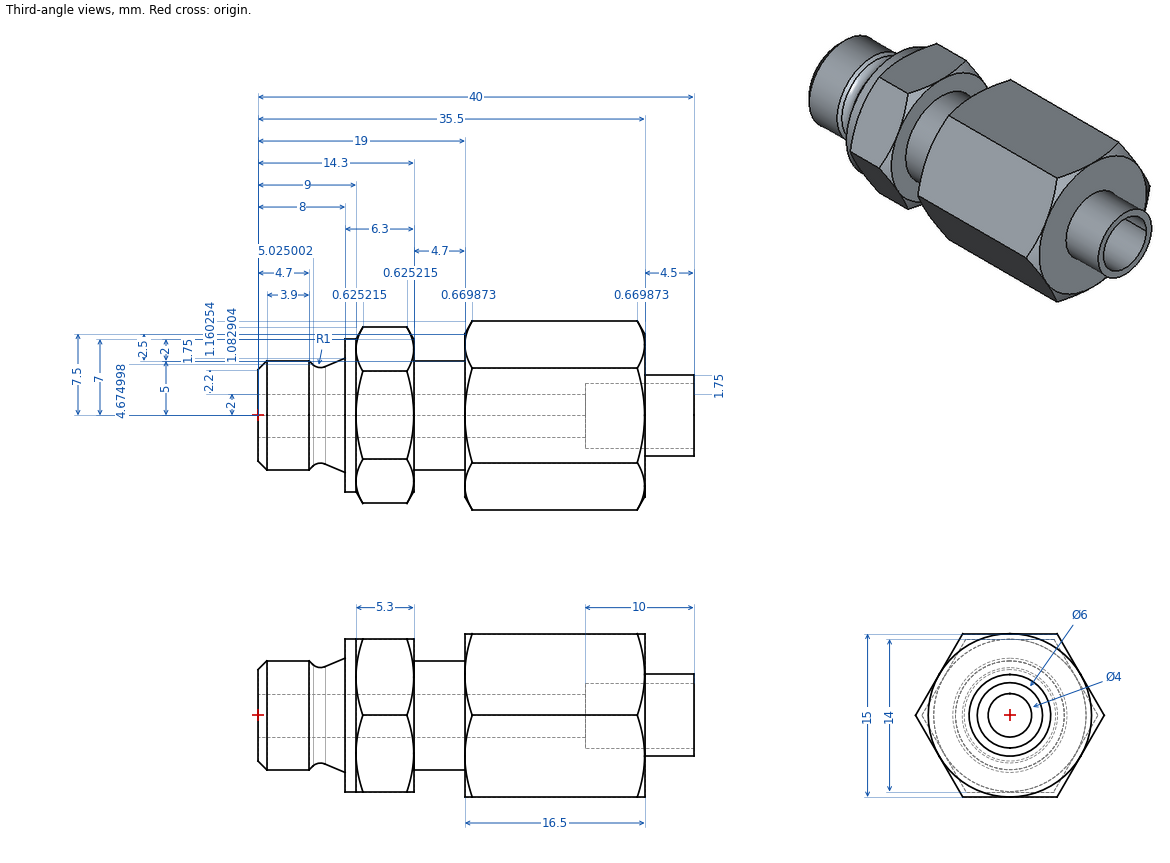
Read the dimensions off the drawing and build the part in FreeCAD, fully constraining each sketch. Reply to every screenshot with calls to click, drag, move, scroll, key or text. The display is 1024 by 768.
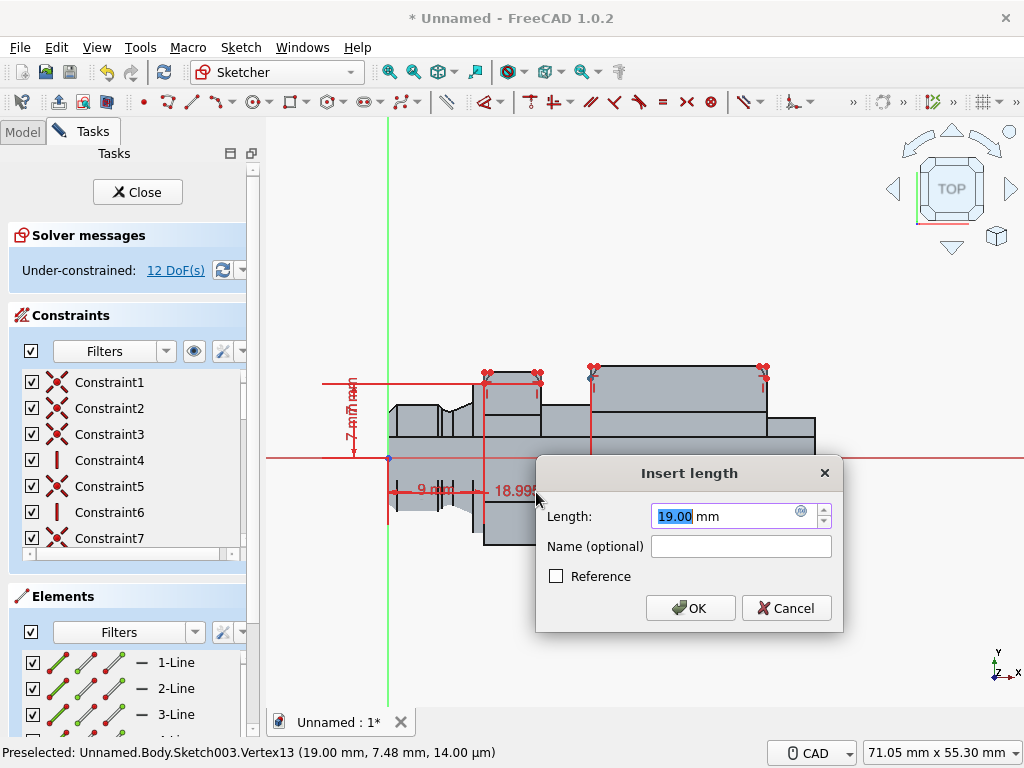
text(19)
key(Return)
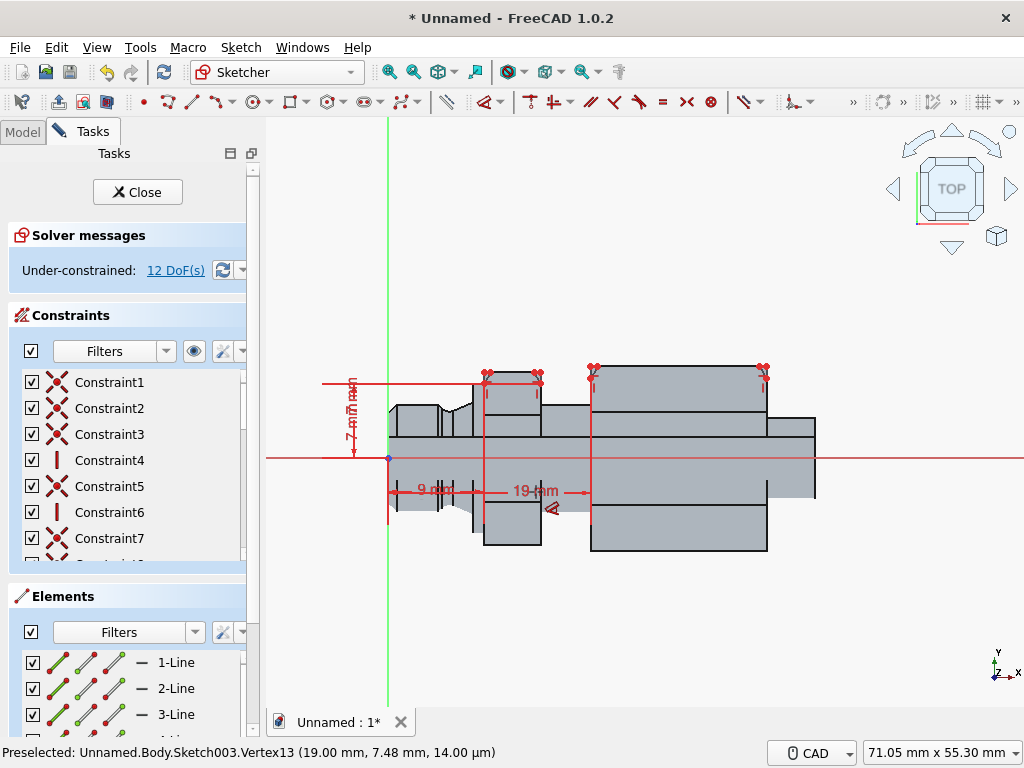
click(591, 379)
click(625, 419)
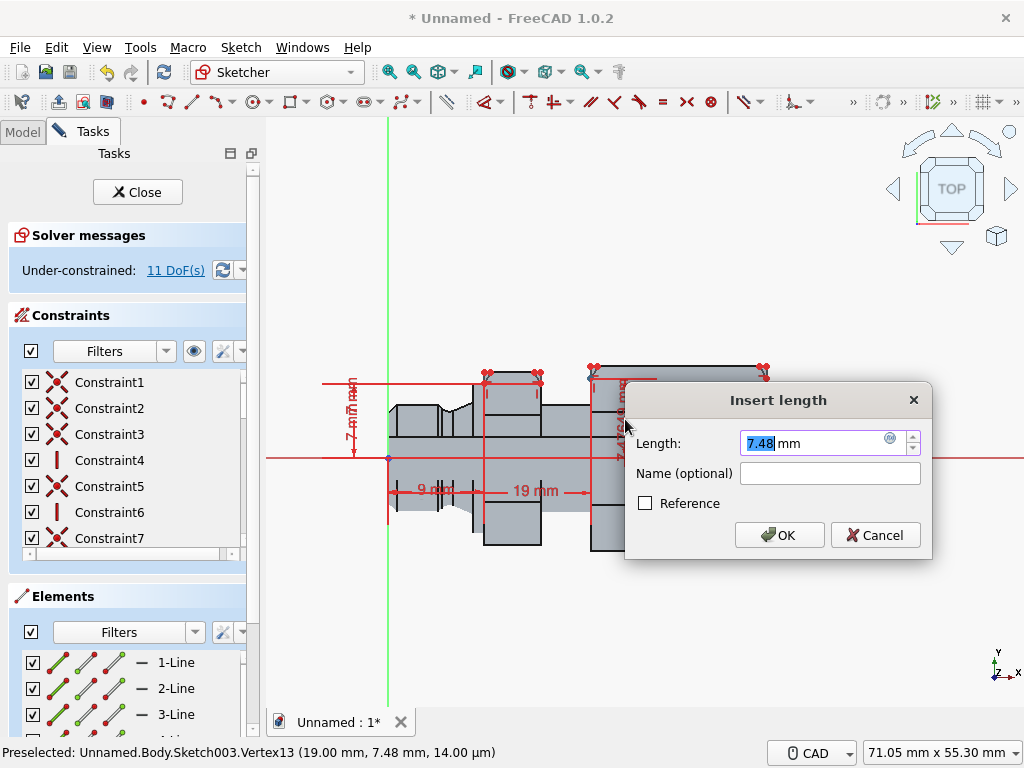
text(7.5)
key(Return)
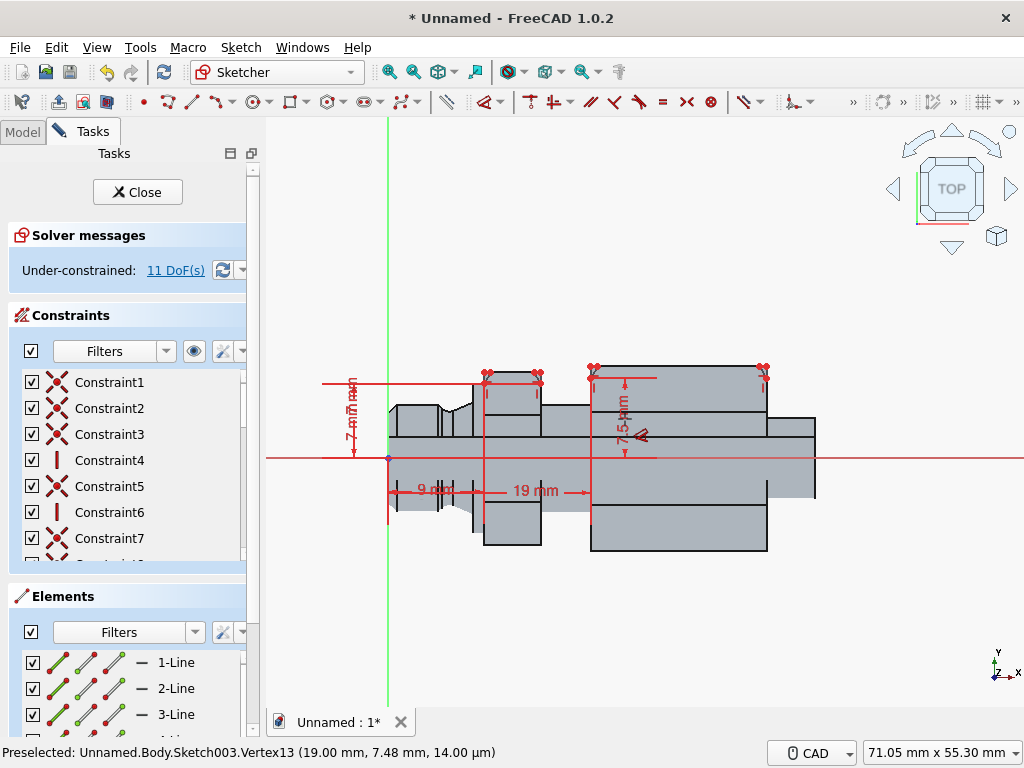
click(767, 379)
click(801, 419)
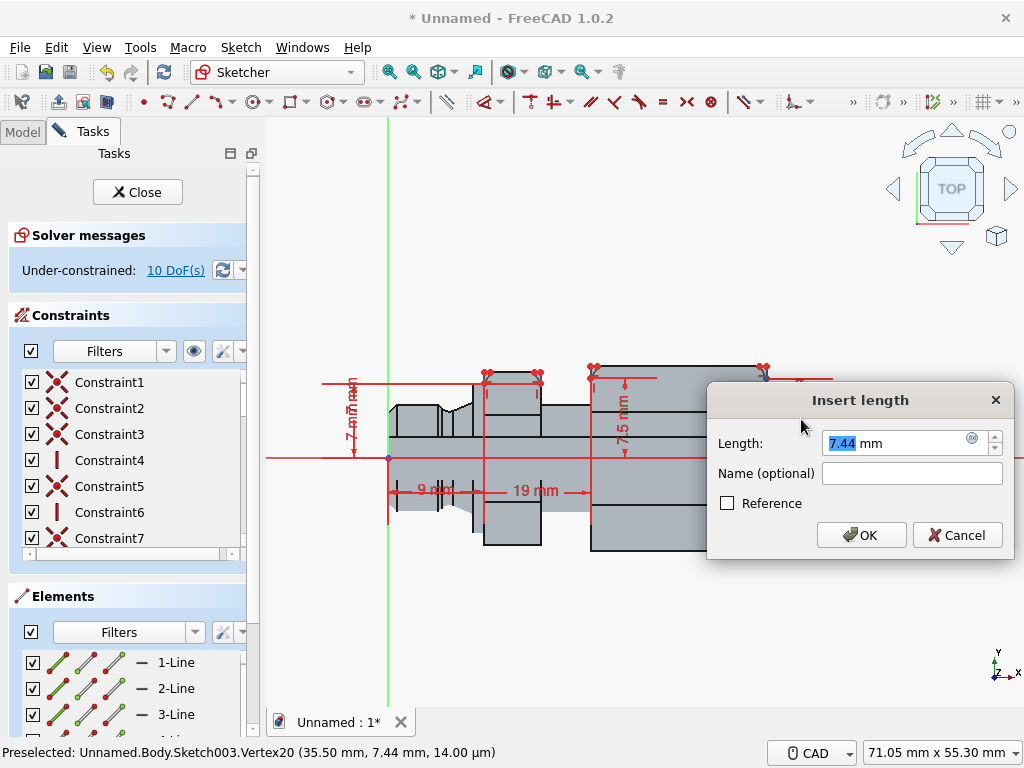
text(7.5)
key(Return)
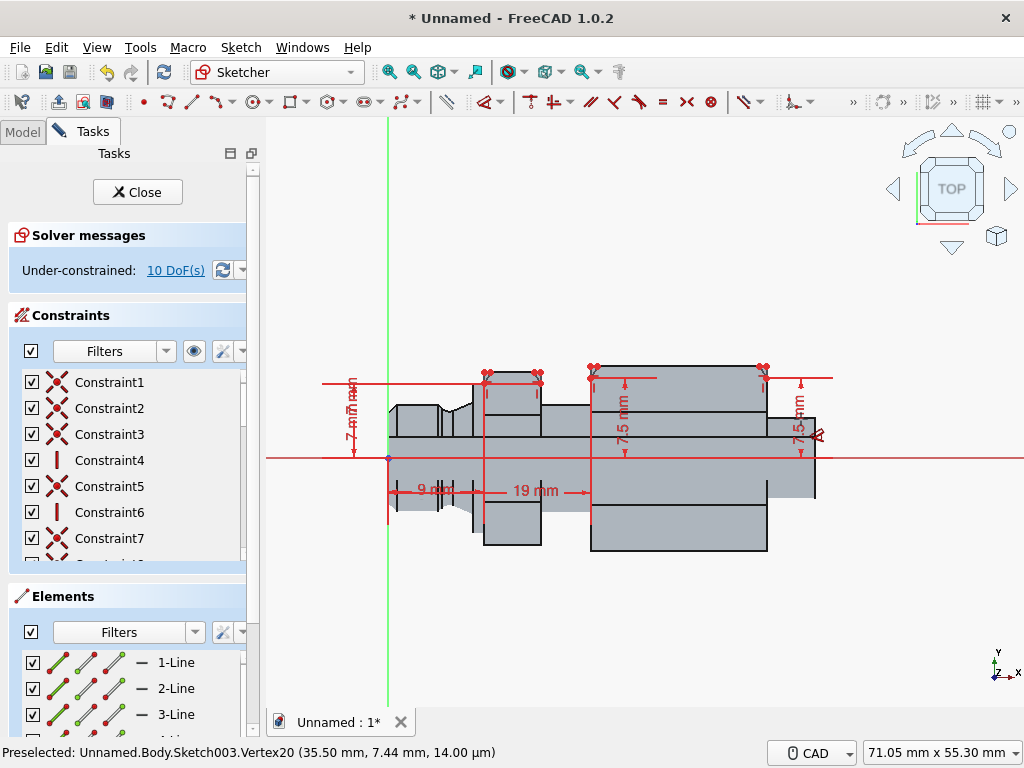
click(541, 384)
click(464, 350)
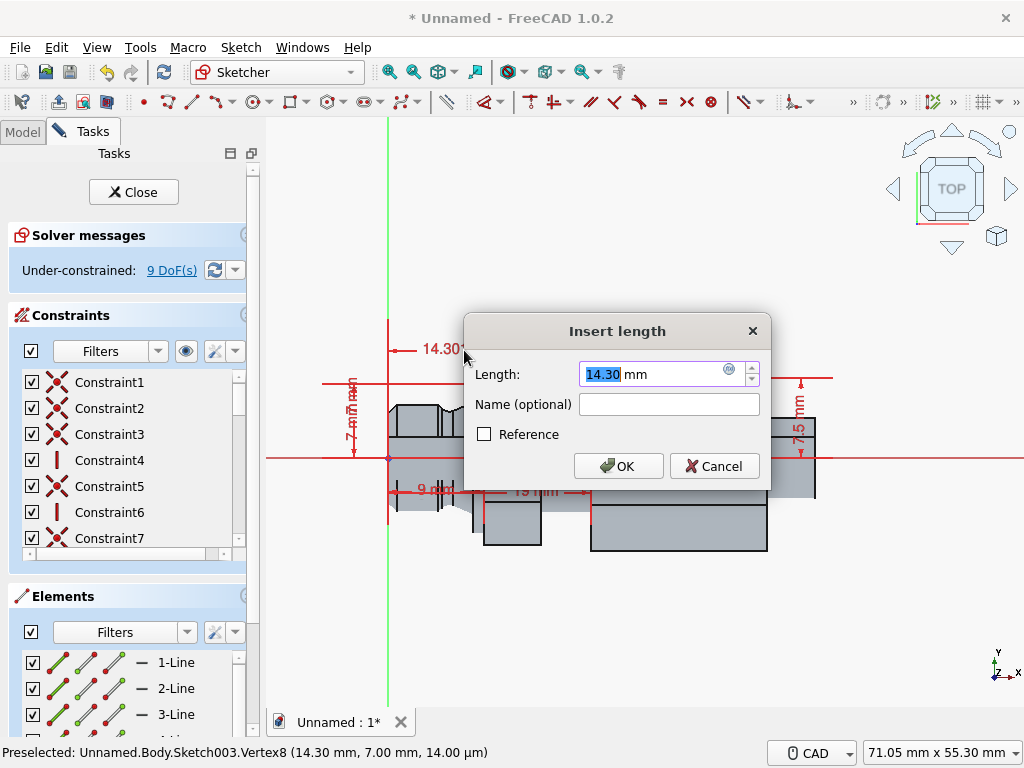
text(14.3)
key(Return)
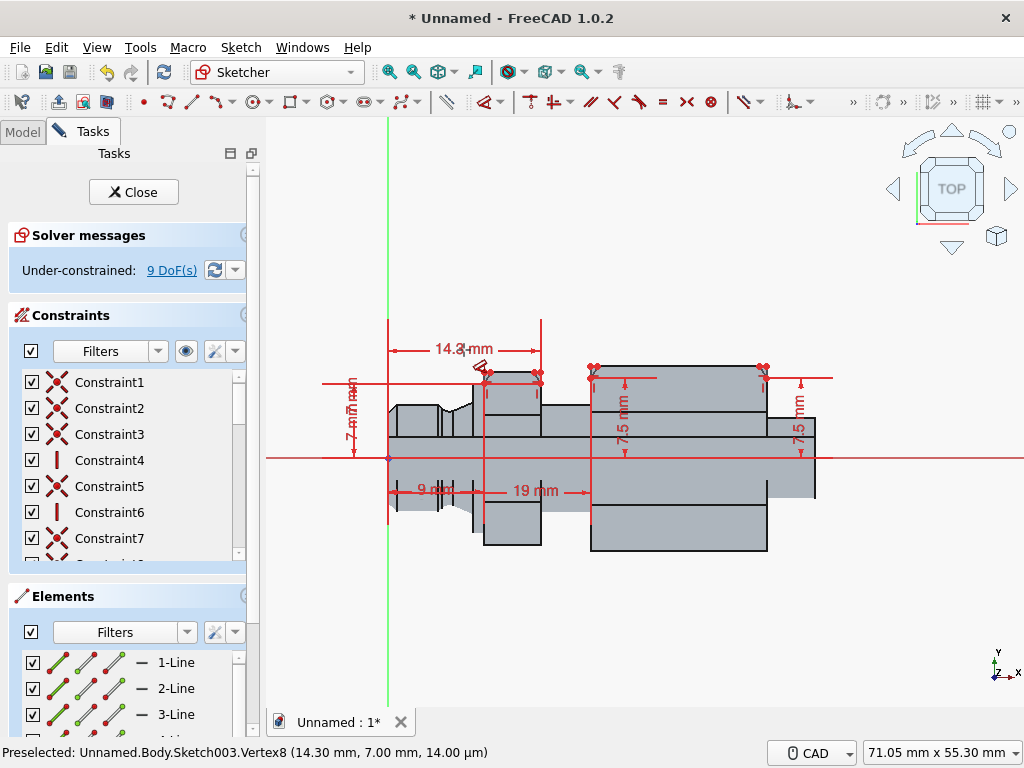
click(767, 378)
click(665, 492)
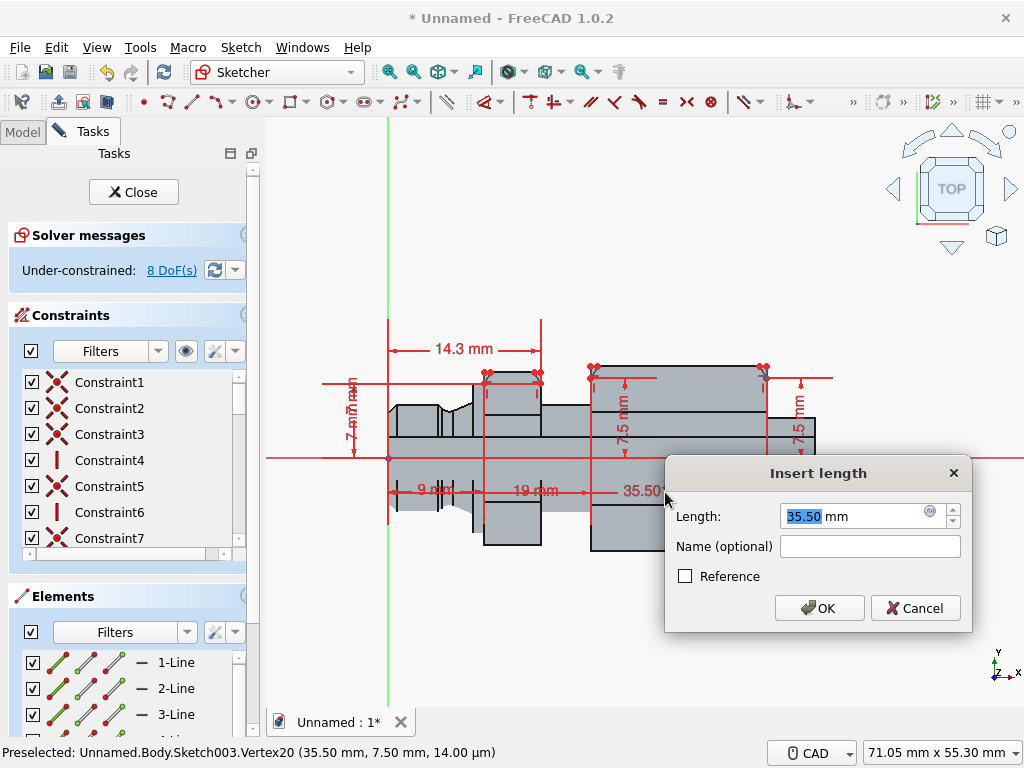
text(35.5)
key(Return)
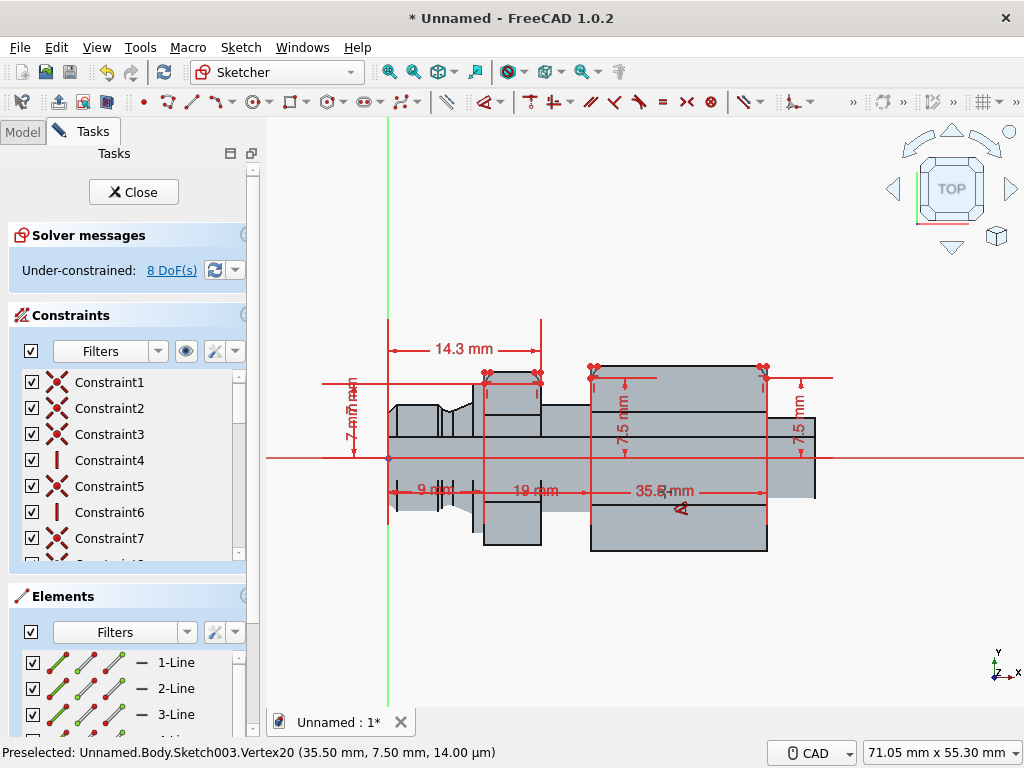
scroll(487, 373, up, 9)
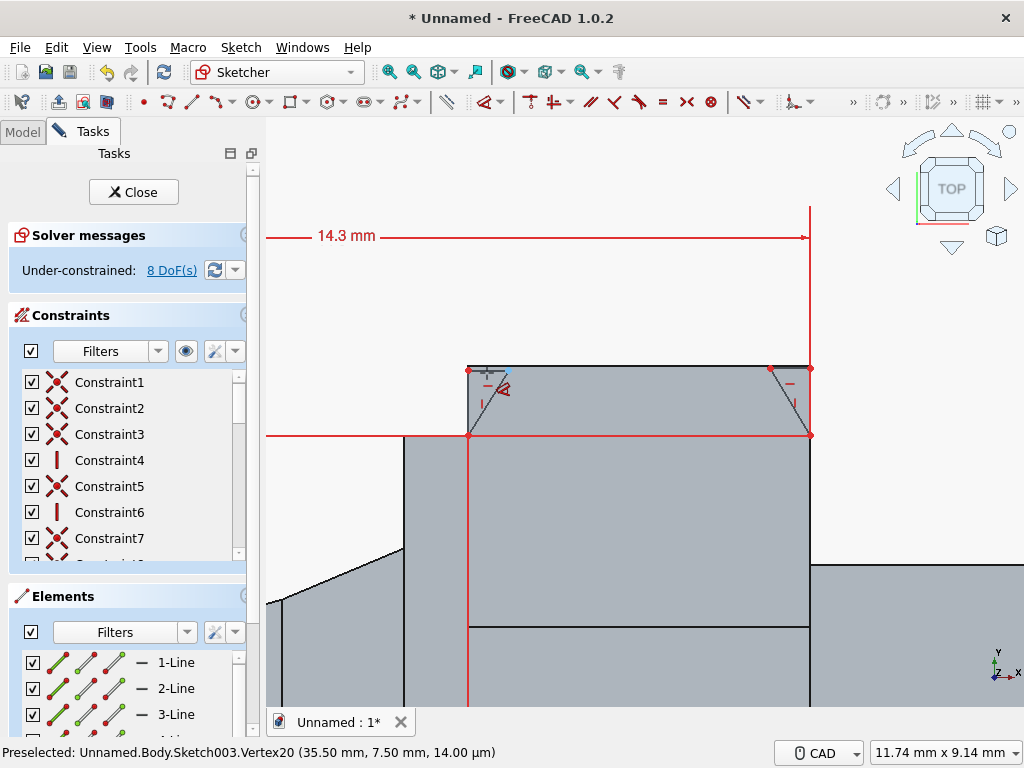
click(489, 371)
click(489, 337)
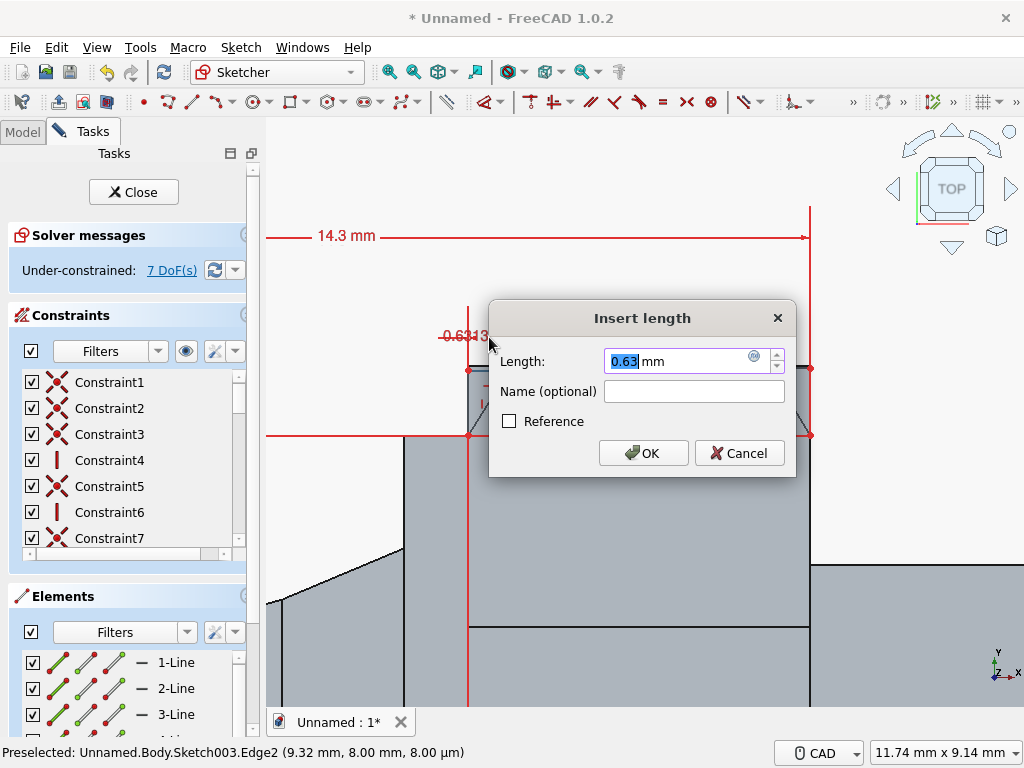
text(0.625215)
key(Return)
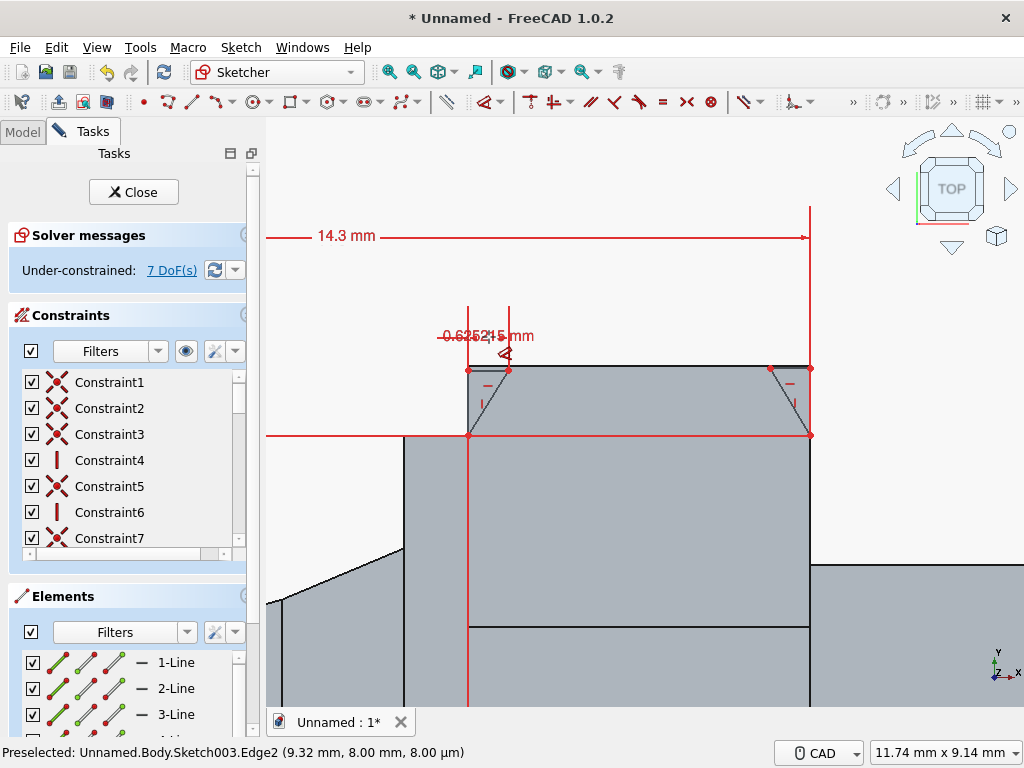
click(468, 390)
click(434, 403)